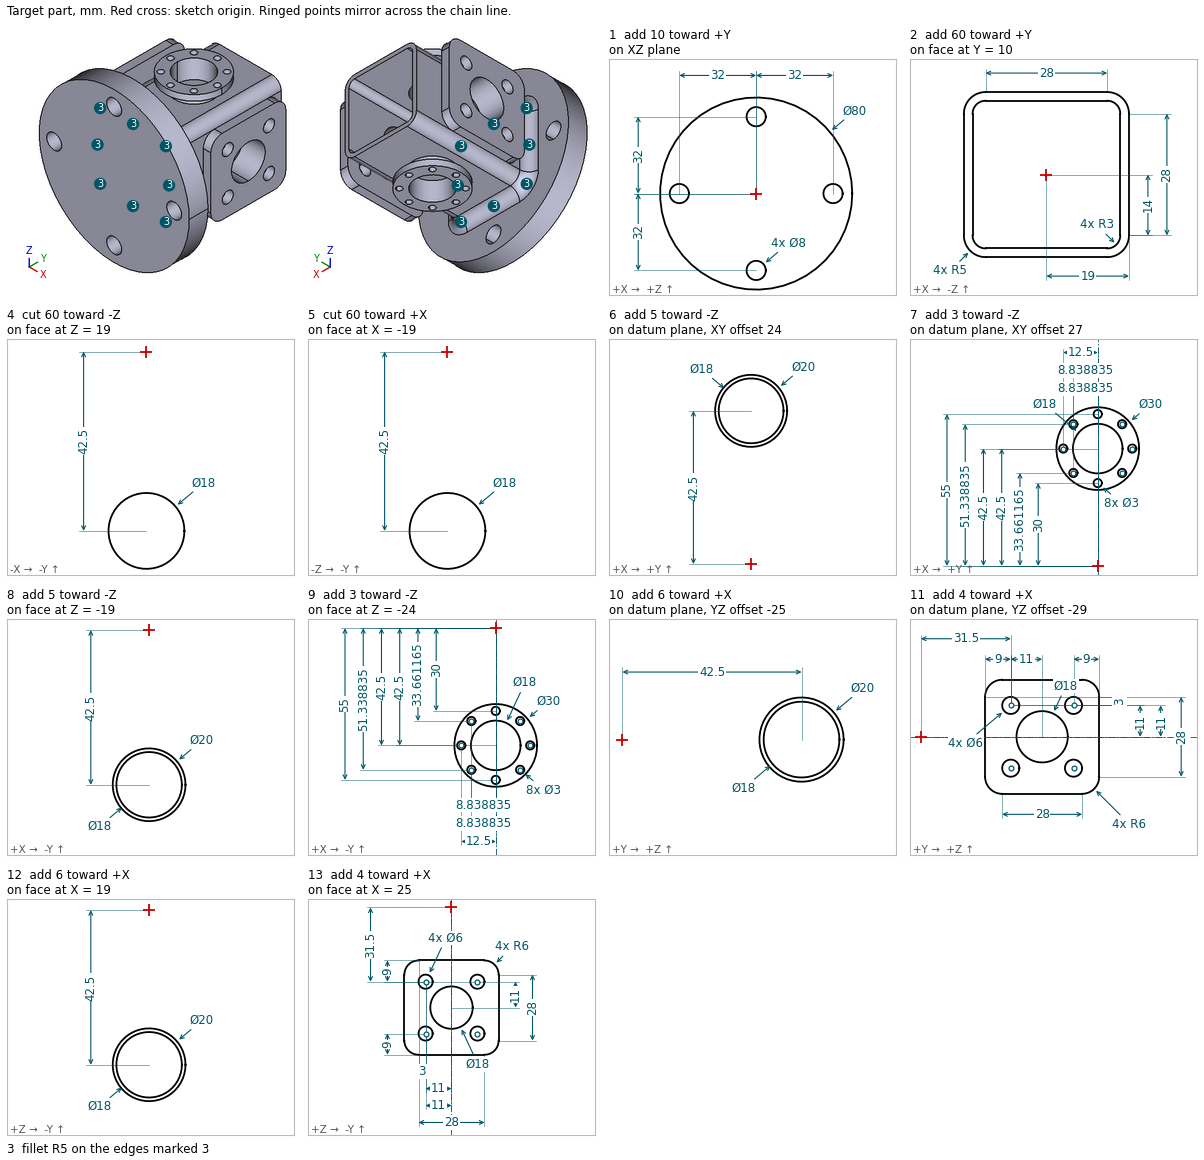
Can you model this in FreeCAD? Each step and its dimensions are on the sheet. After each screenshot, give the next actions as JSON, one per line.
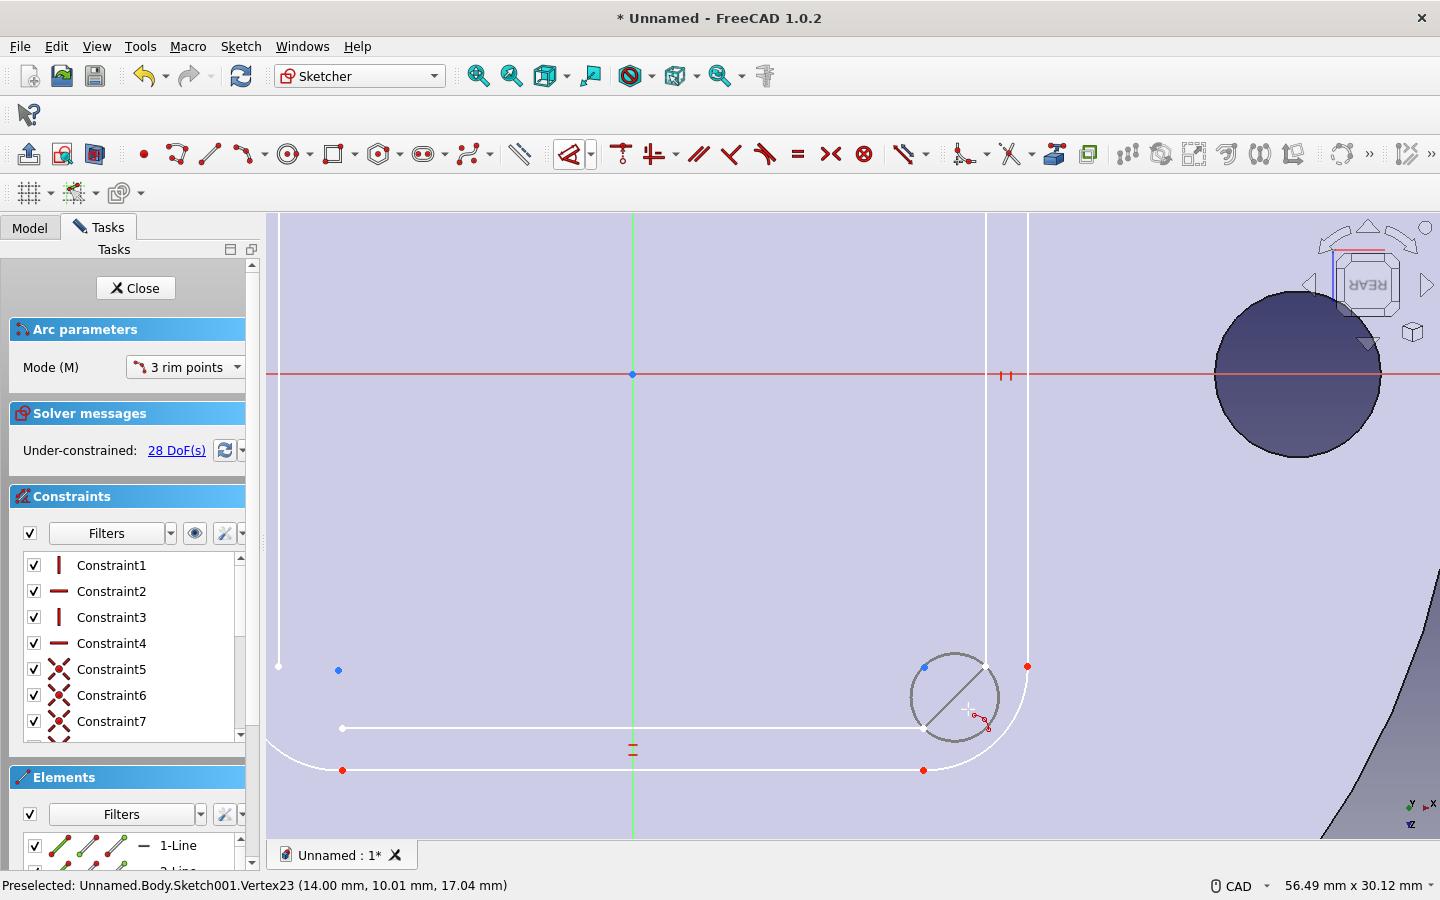
{"action": "left_click", "coordinate": [968, 709]}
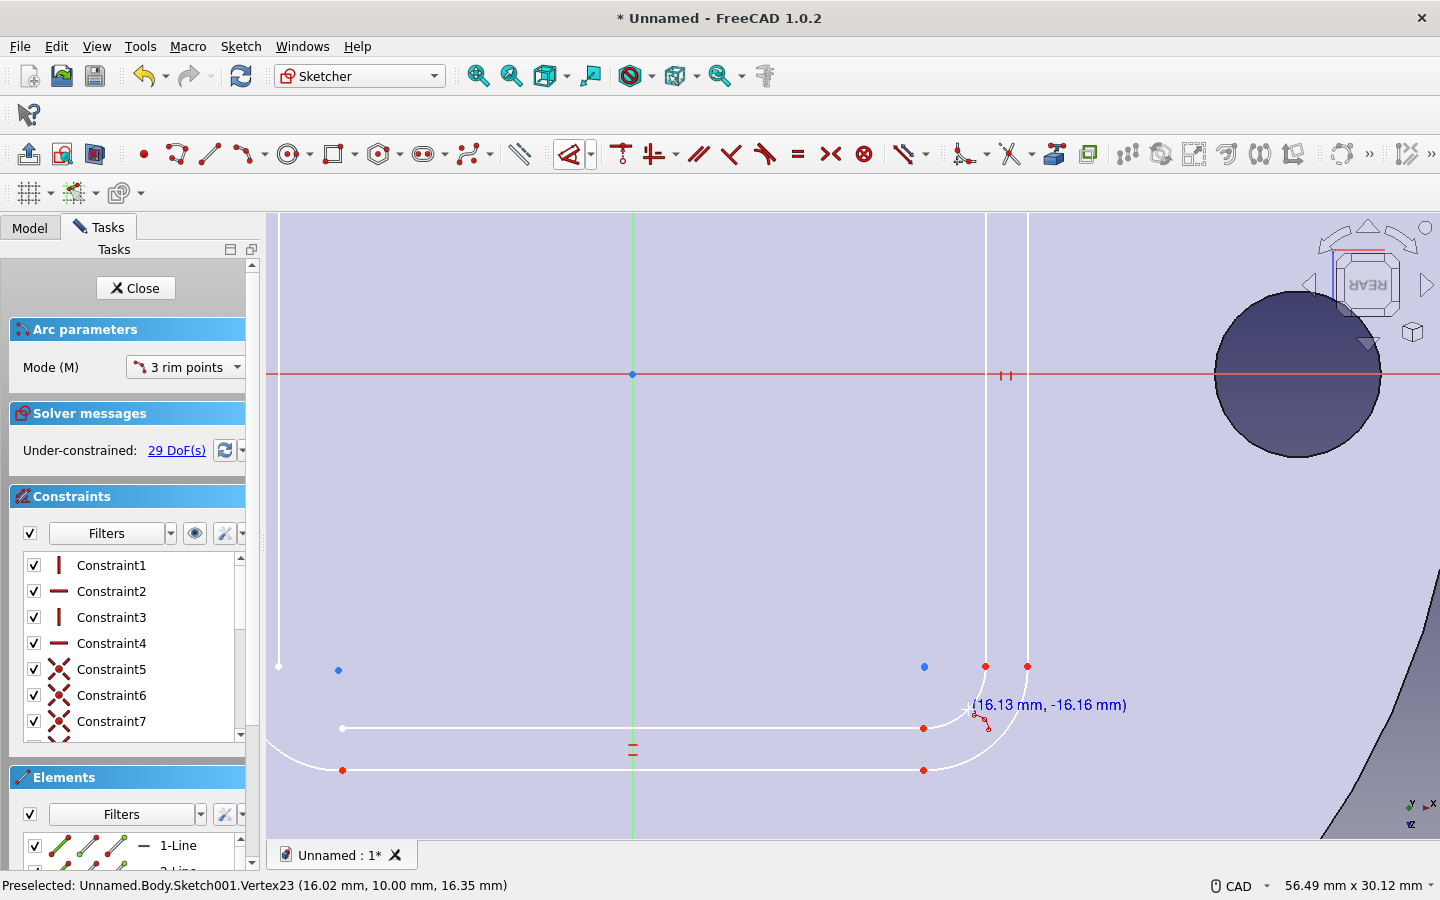
{"action": "left_click", "coordinate": [343, 728]}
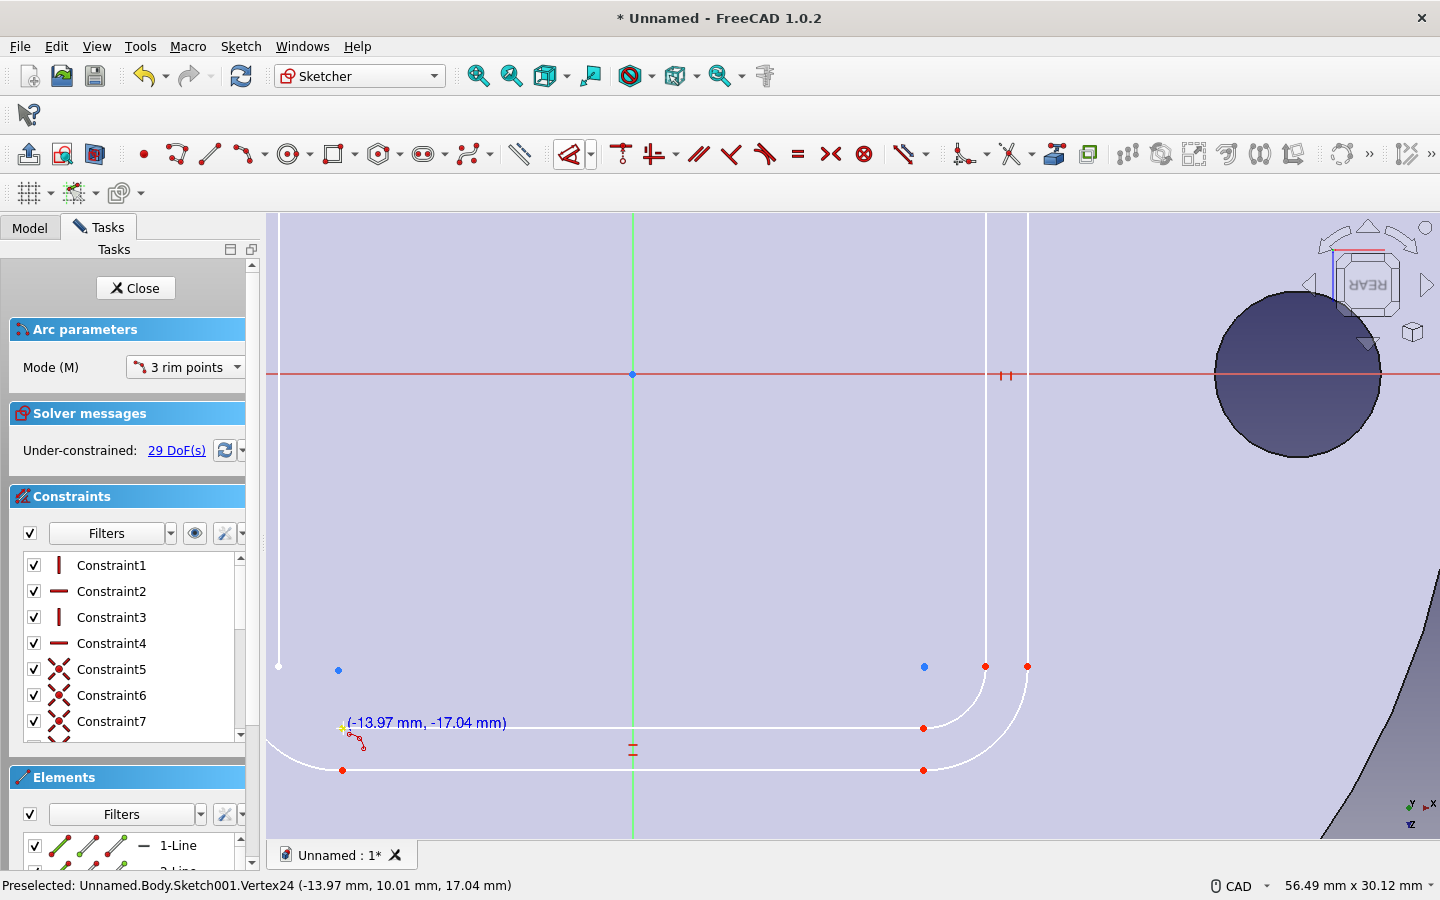
{"action": "scroll", "coordinate": [969, 711], "scroll_direction": "down", "scroll_amount": 3}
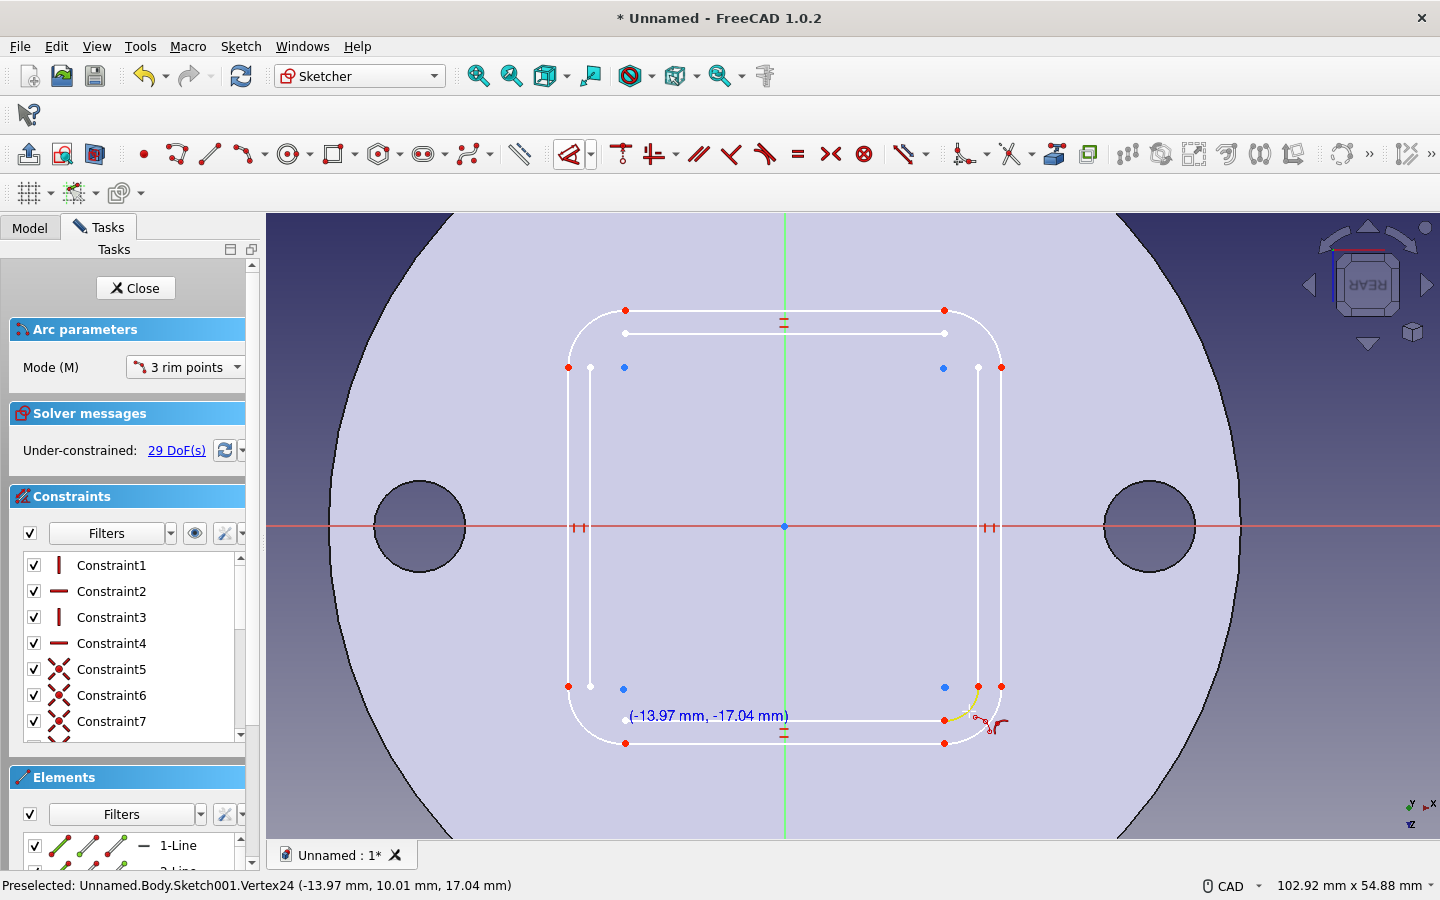
{"action": "left_click", "coordinate": [590, 687]}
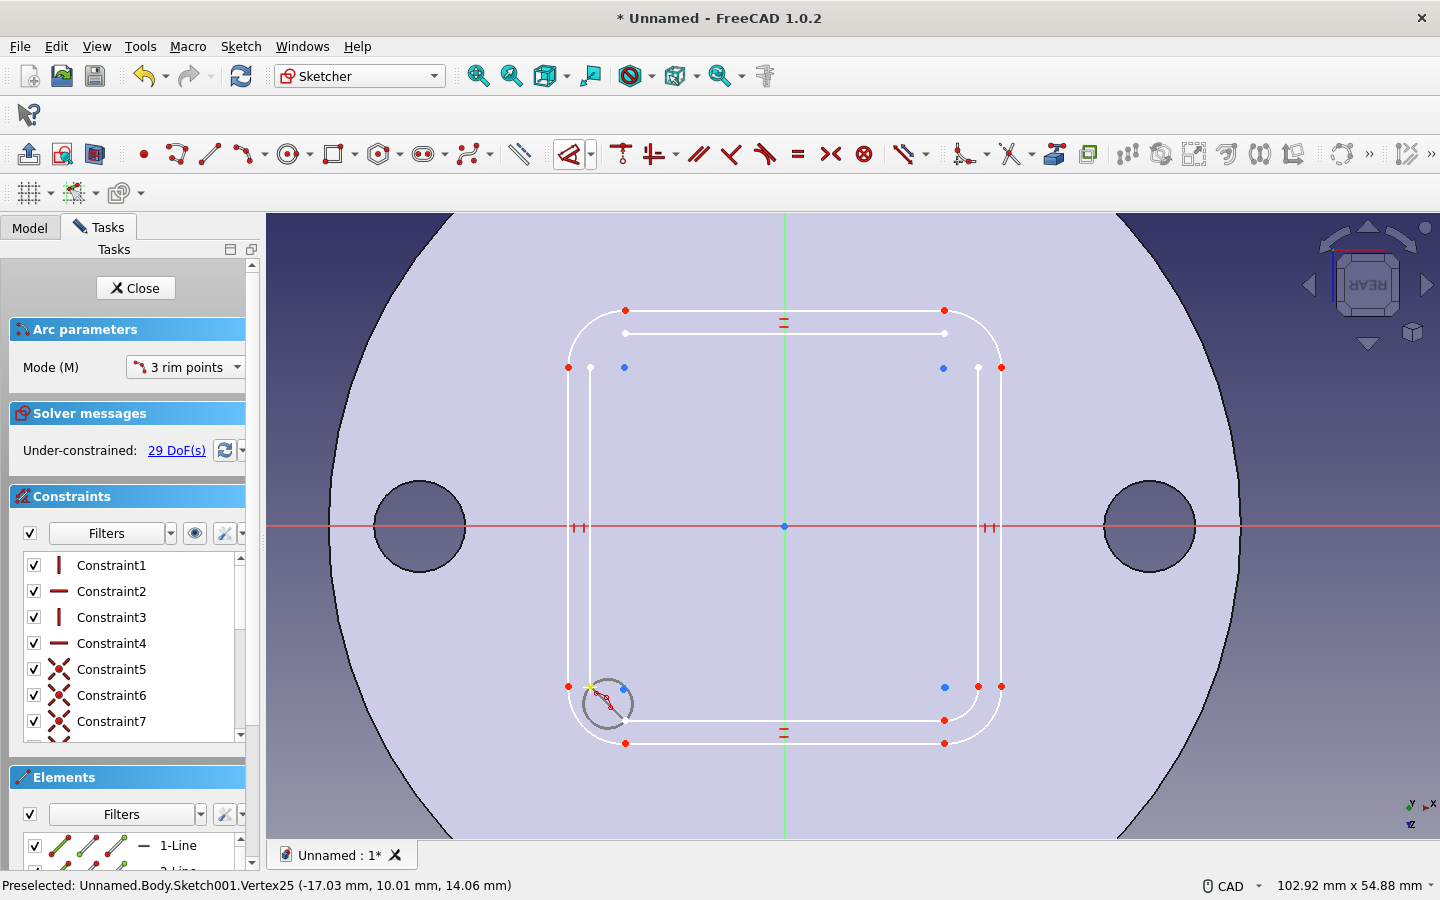
{"action": "scroll", "coordinate": [601, 710], "scroll_direction": "up", "scroll_amount": 3}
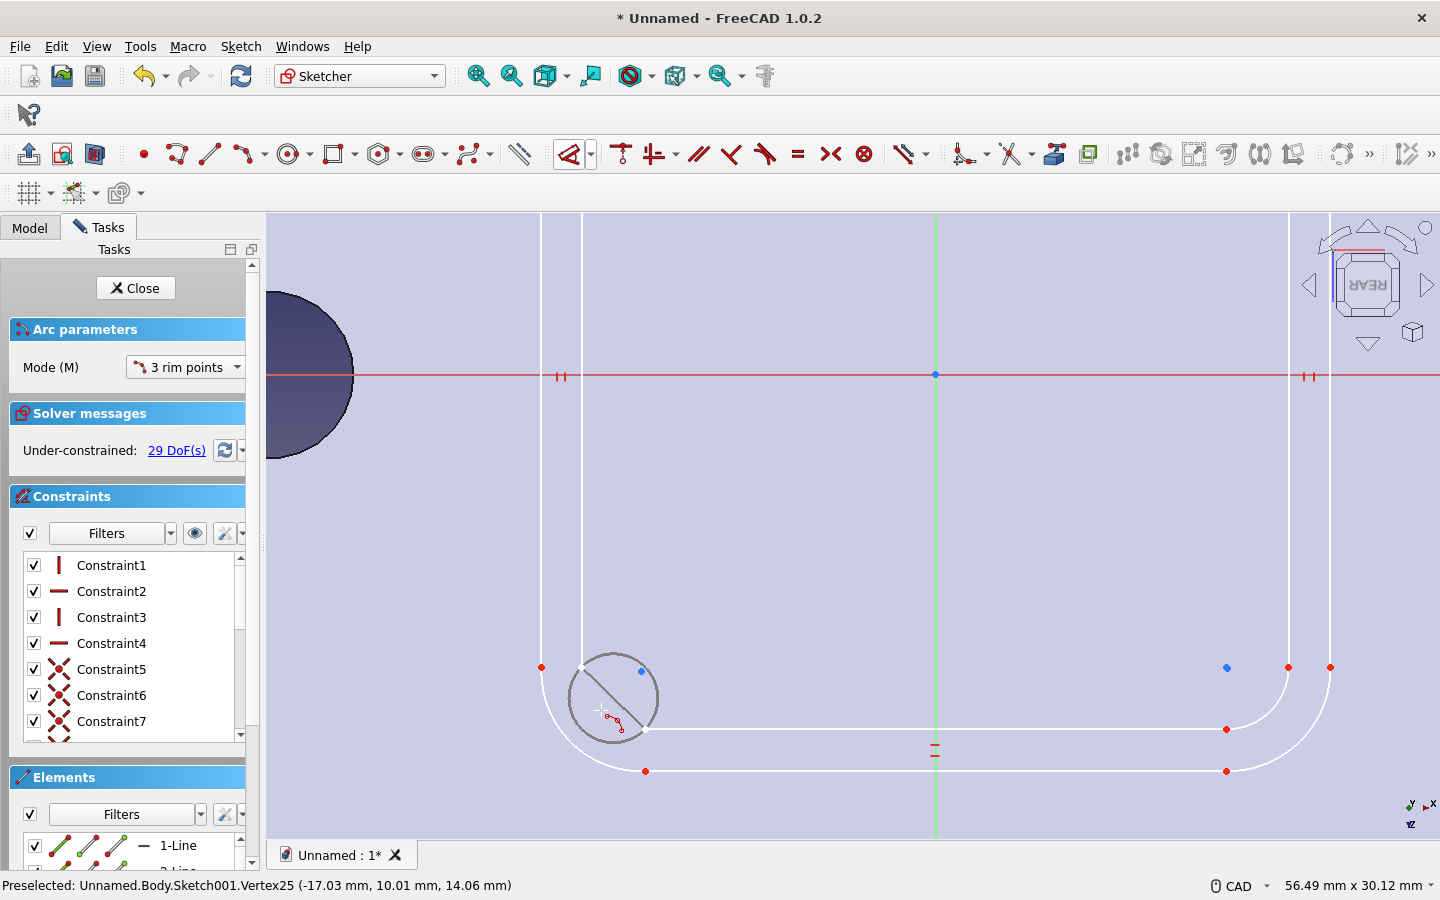
{"action": "left_click", "coordinate": [601, 710]}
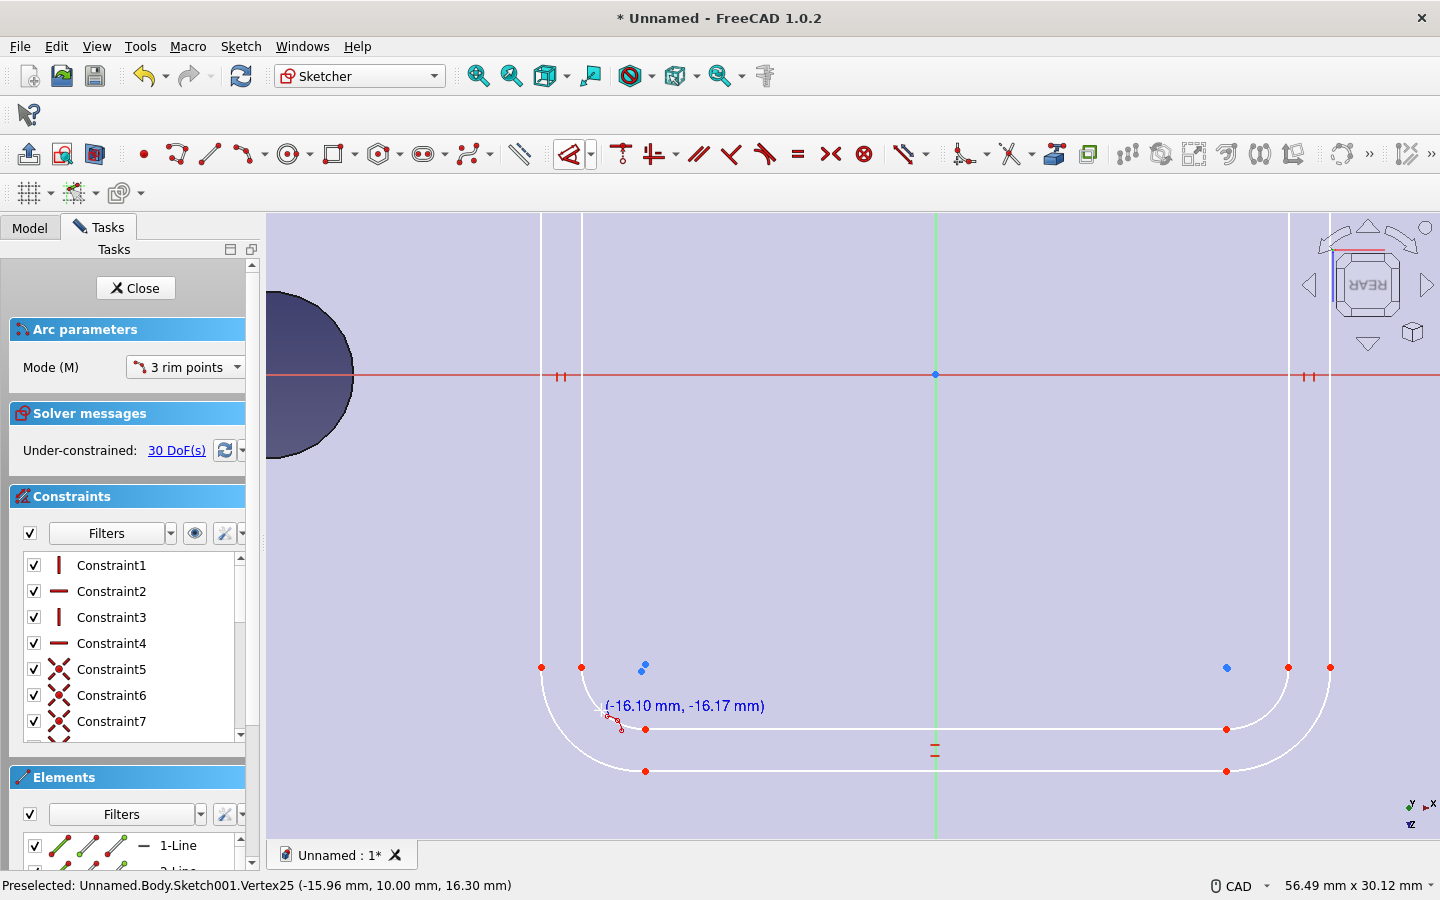
{"action": "scroll", "coordinate": [601, 710], "scroll_direction": "down", "scroll_amount": 3}